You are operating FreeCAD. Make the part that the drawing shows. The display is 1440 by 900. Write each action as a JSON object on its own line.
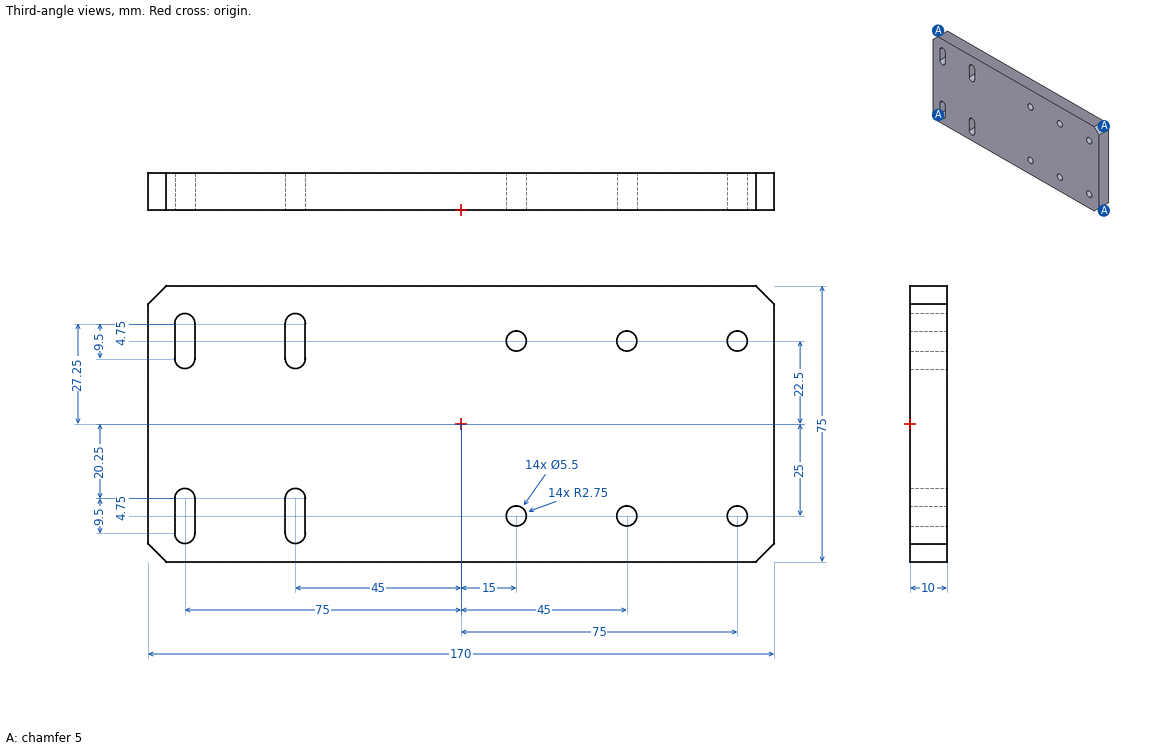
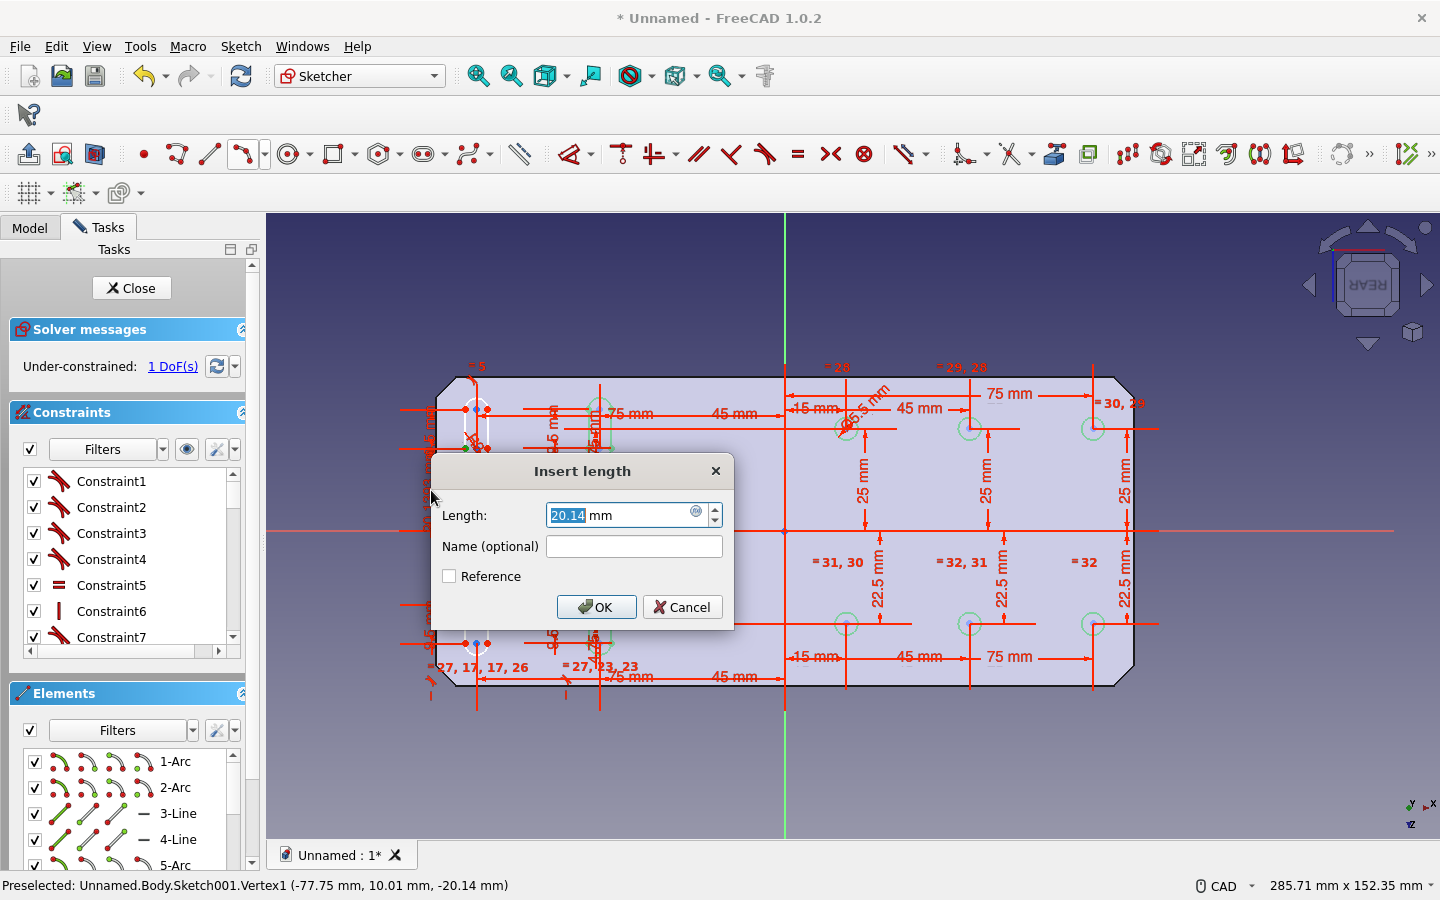
{"action": "type", "text": "20.25"}
{"action": "key", "text": "Return"}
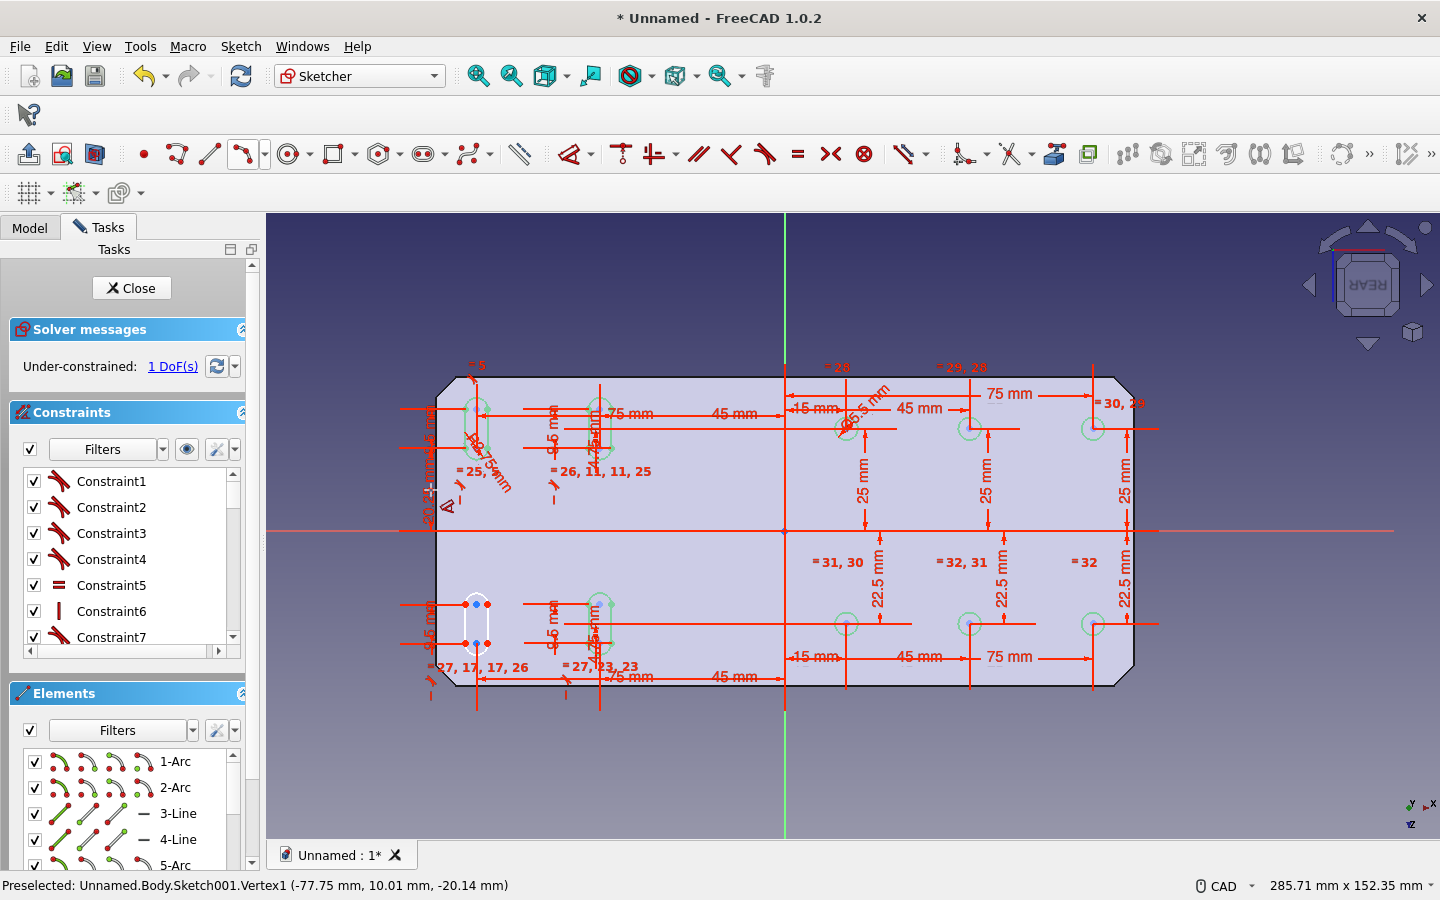
{"action": "left_click", "coordinate": [465, 644]}
{"action": "left_click", "coordinate": [431, 588]}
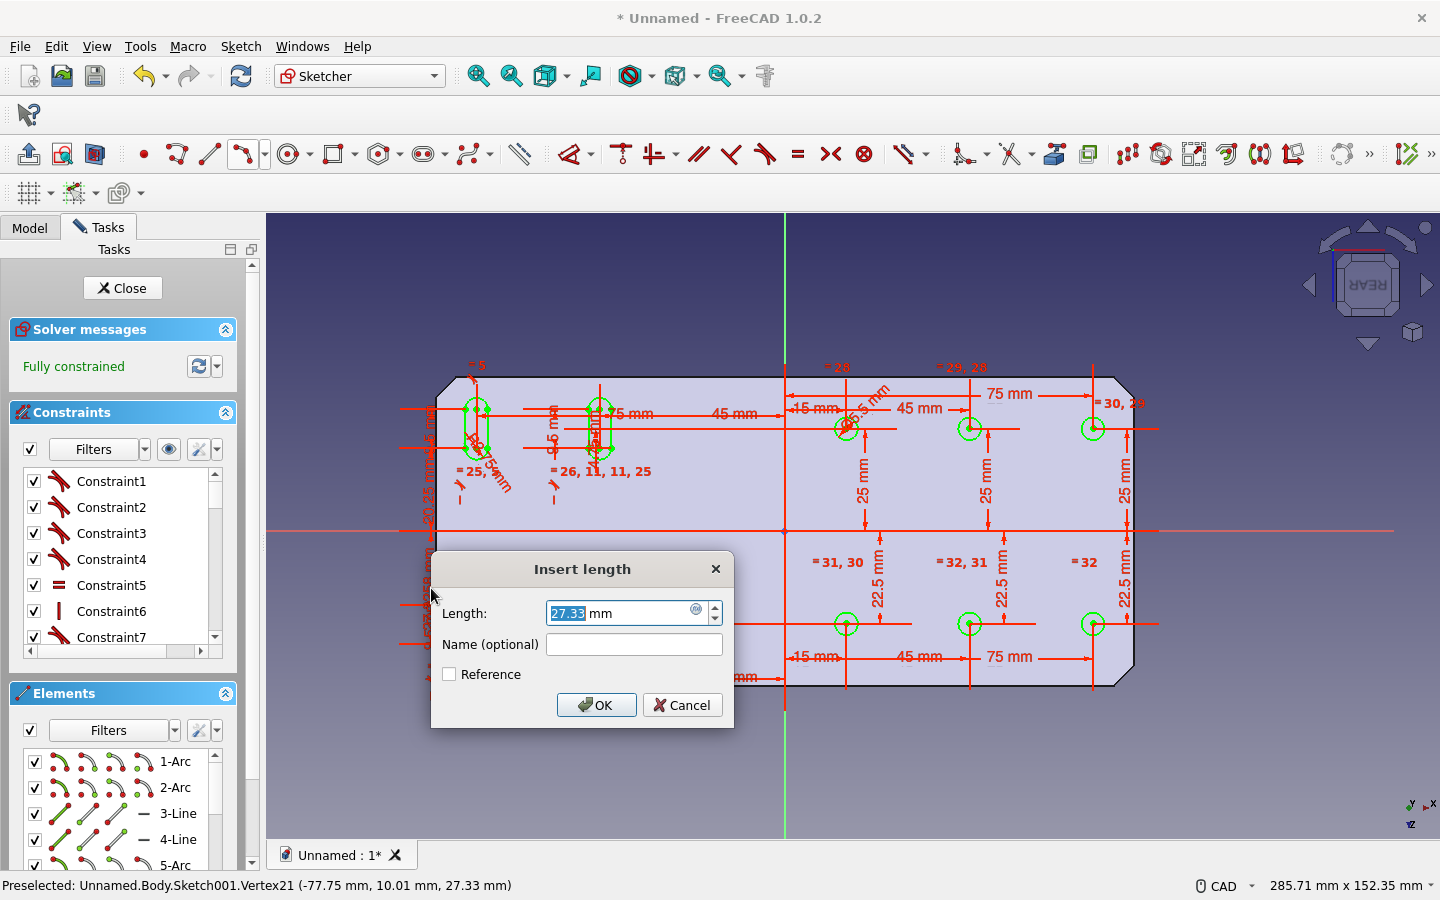
{"action": "type", "text": "27.25"}
{"action": "key", "text": "Return"}
{"action": "key", "text": "Escape"}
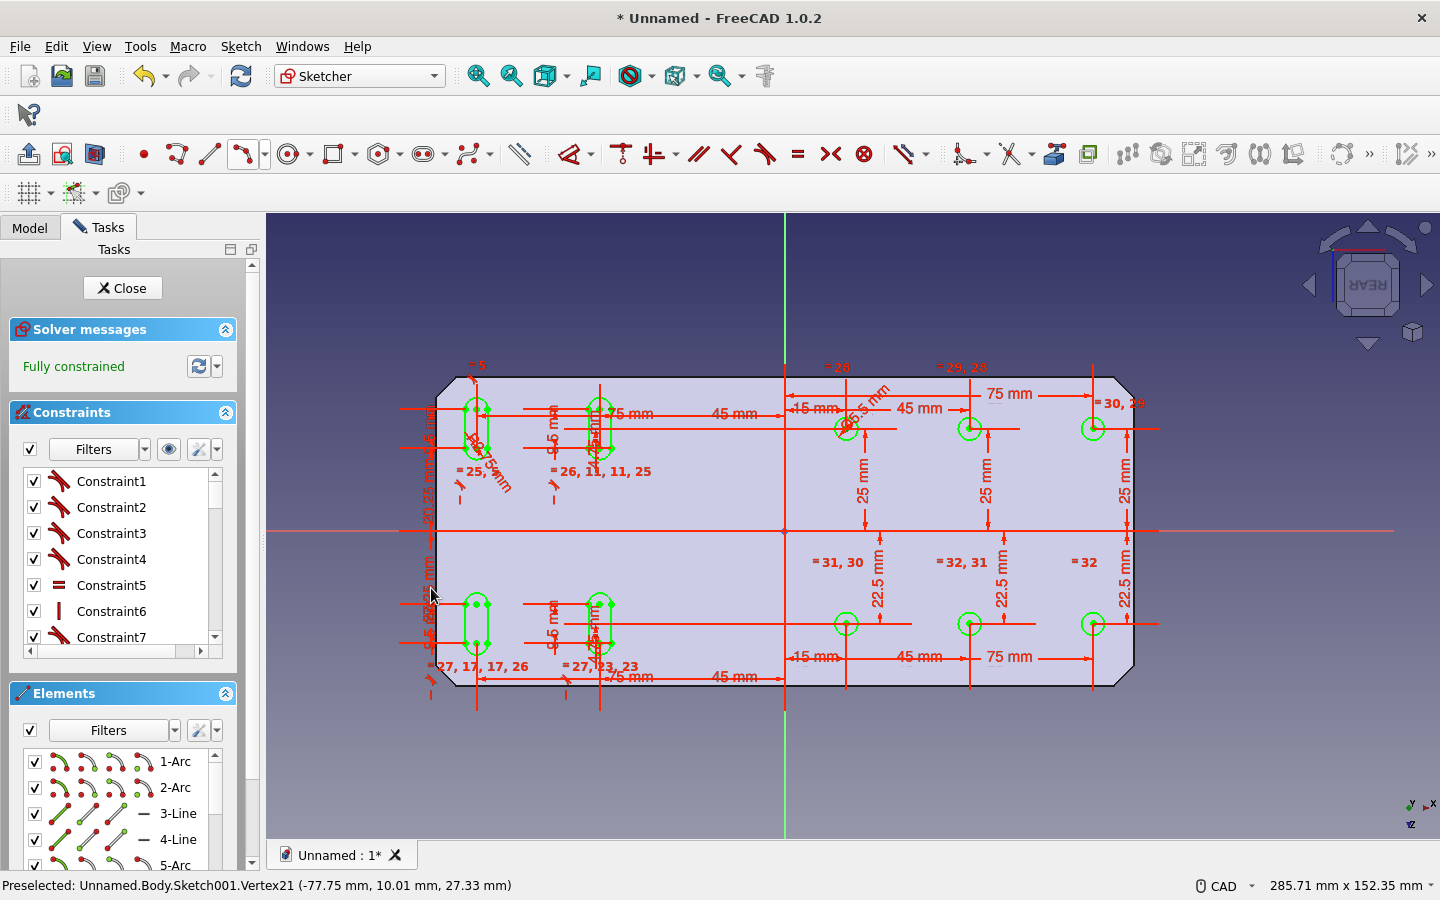
{"action": "left_click", "coordinate": [123, 288]}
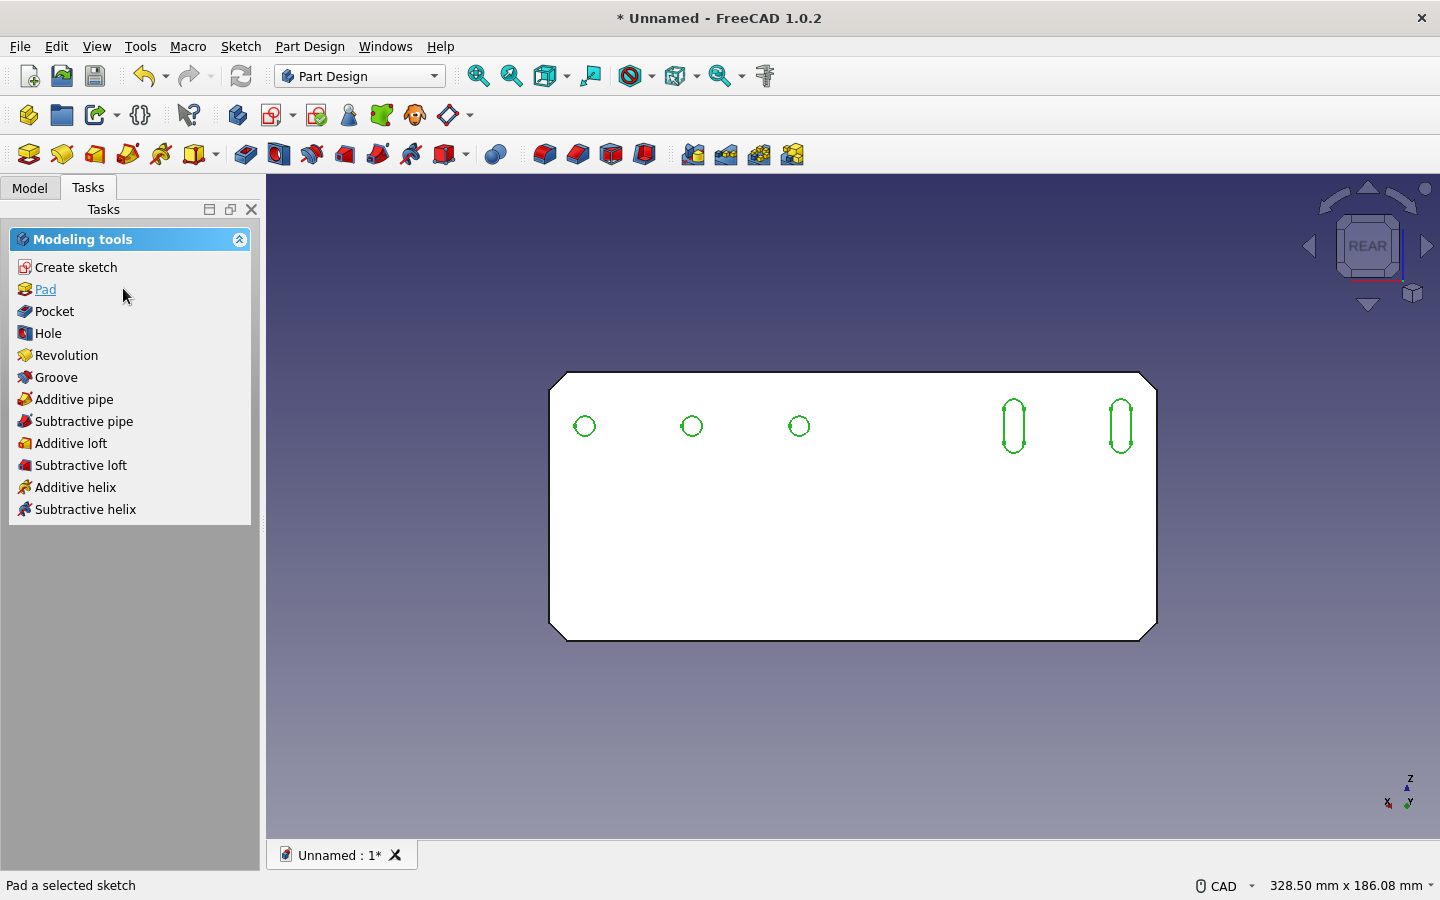
{"action": "left_click", "coordinate": [246, 154]}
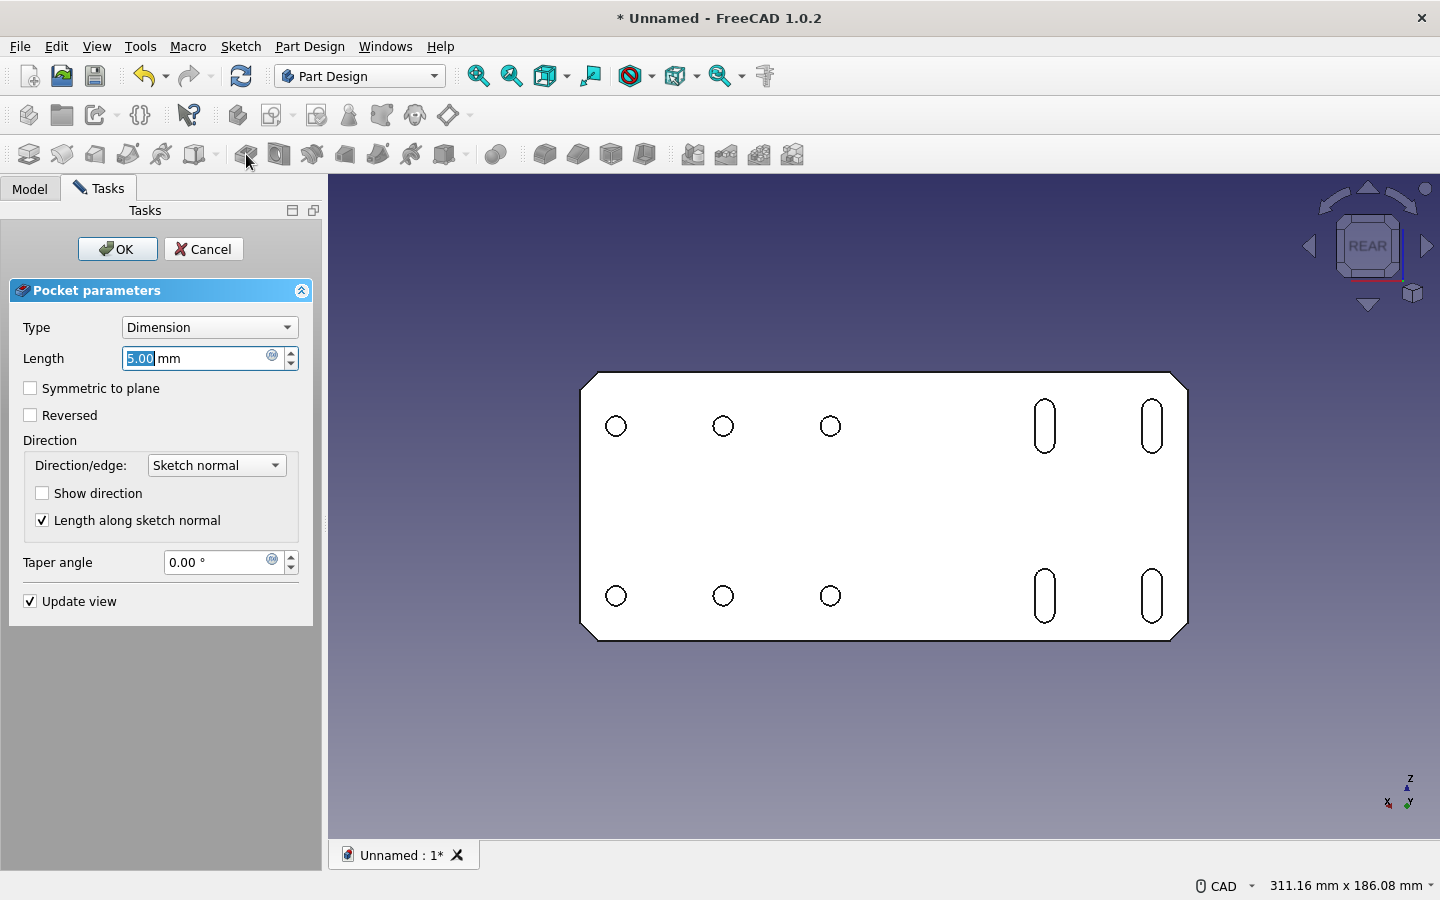
{"action": "type", "text": "15"}
{"action": "key", "text": "Tab"}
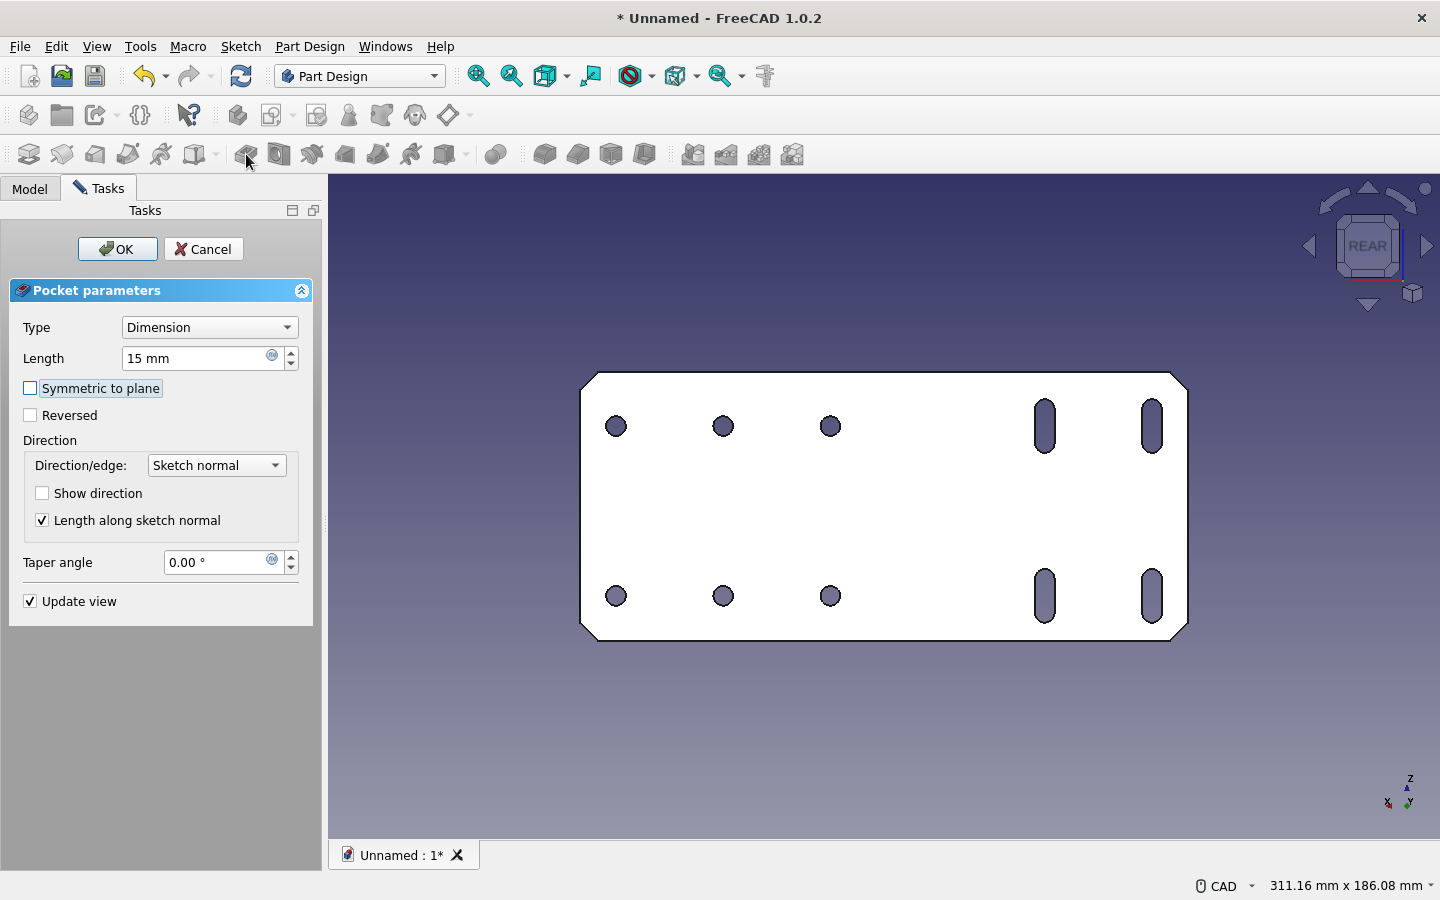
{"action": "left_click", "coordinate": [118, 249]}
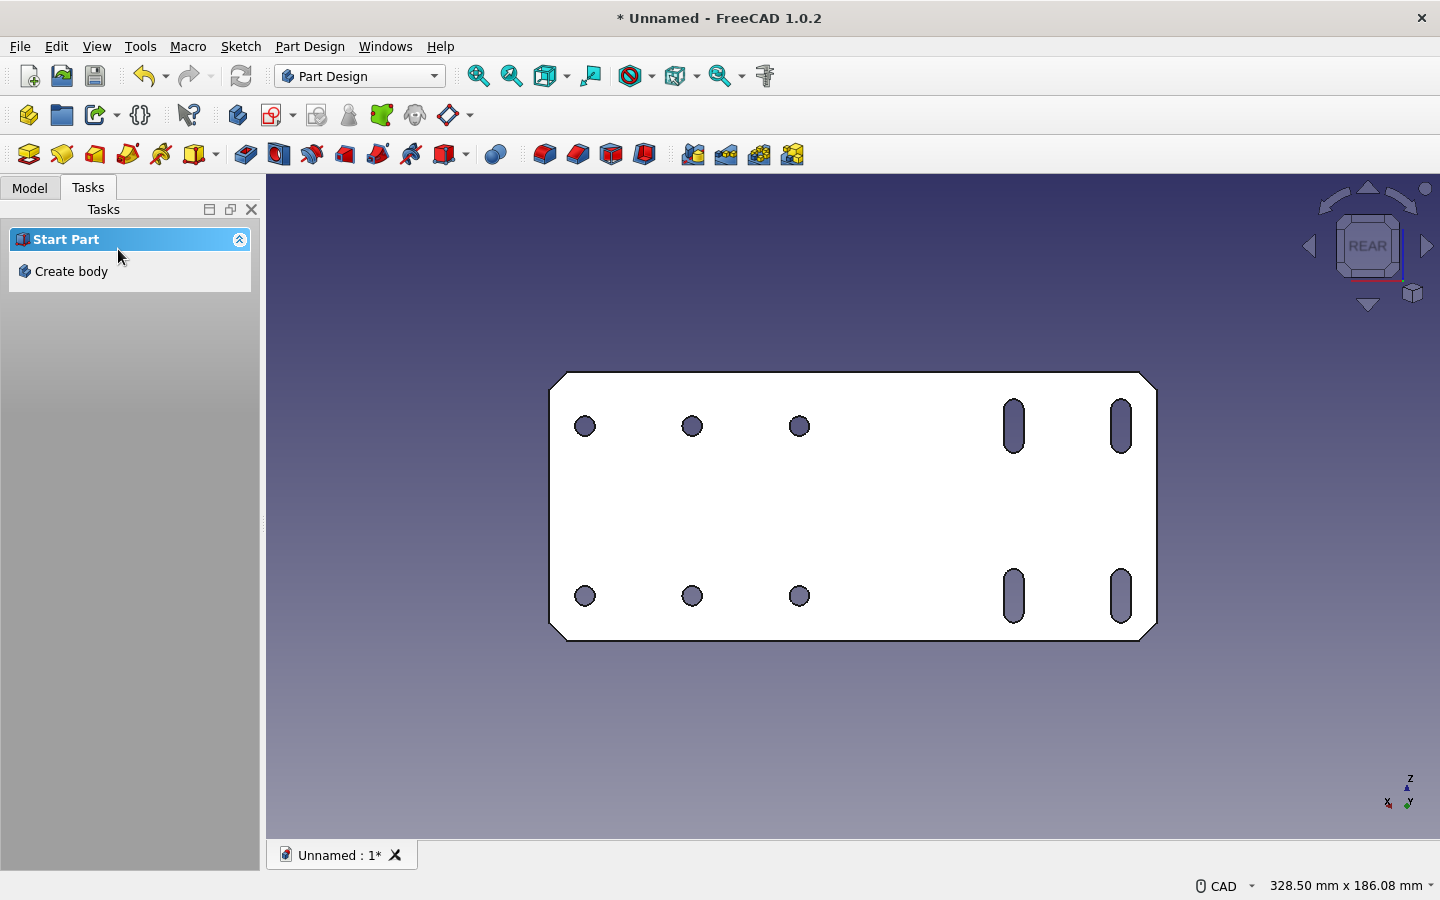
{"action": "key", "text": "0"}